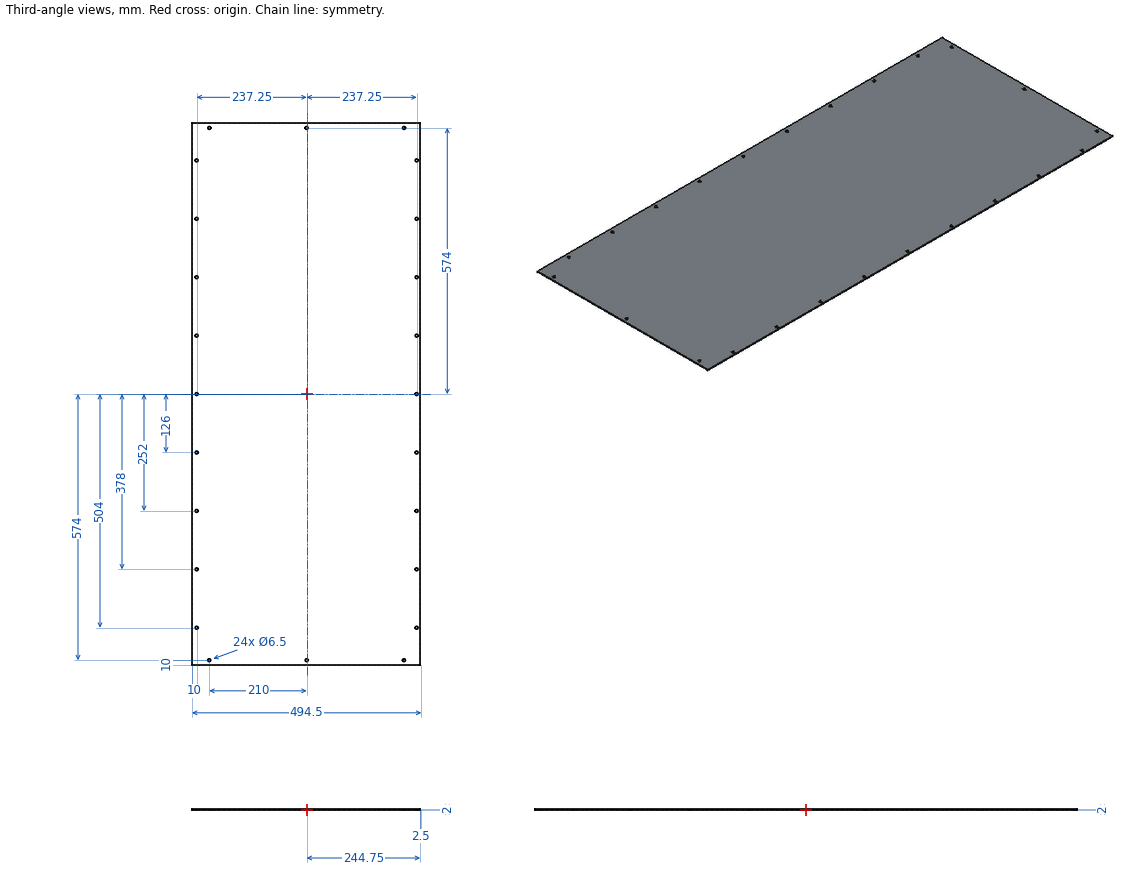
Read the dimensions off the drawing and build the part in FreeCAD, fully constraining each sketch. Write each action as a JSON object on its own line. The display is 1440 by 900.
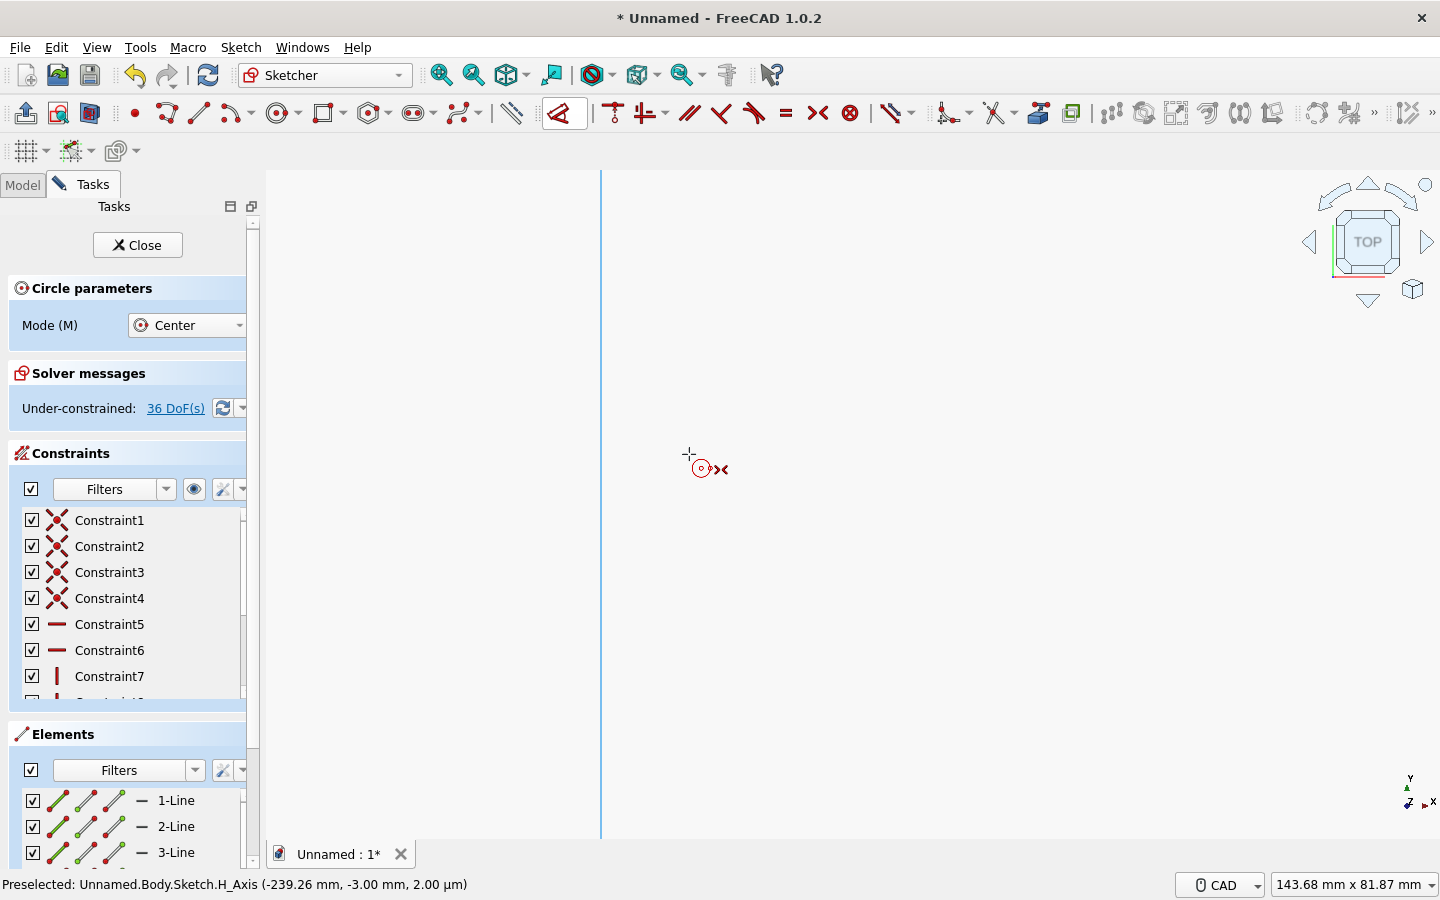
{"action": "scroll", "coordinate": [689, 454], "scroll_direction": "down", "scroll_amount": 15}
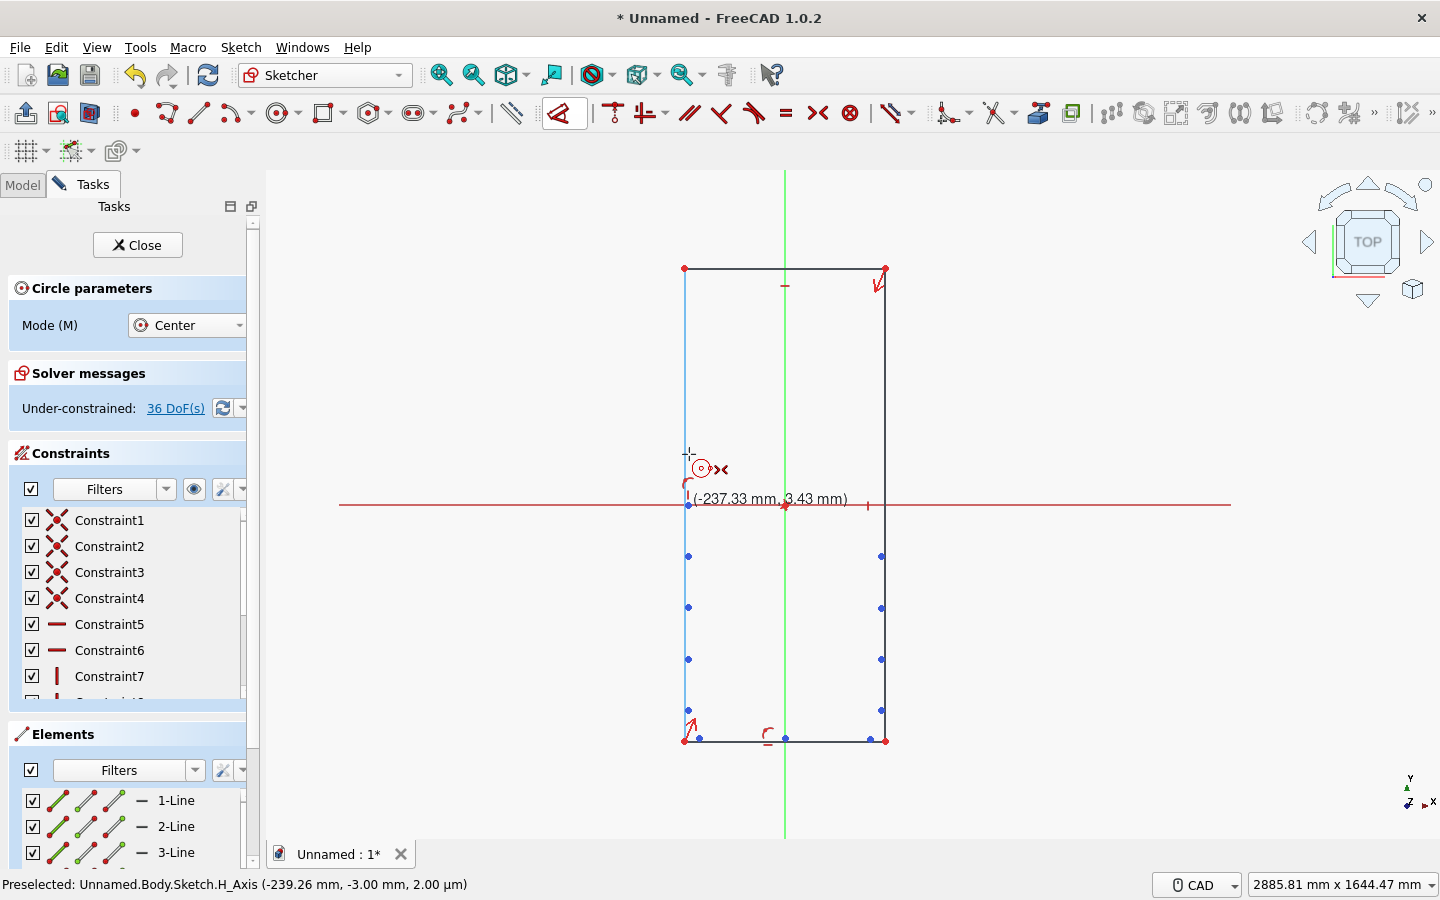
{"action": "scroll", "coordinate": [689, 454], "scroll_direction": "up", "scroll_amount": 7}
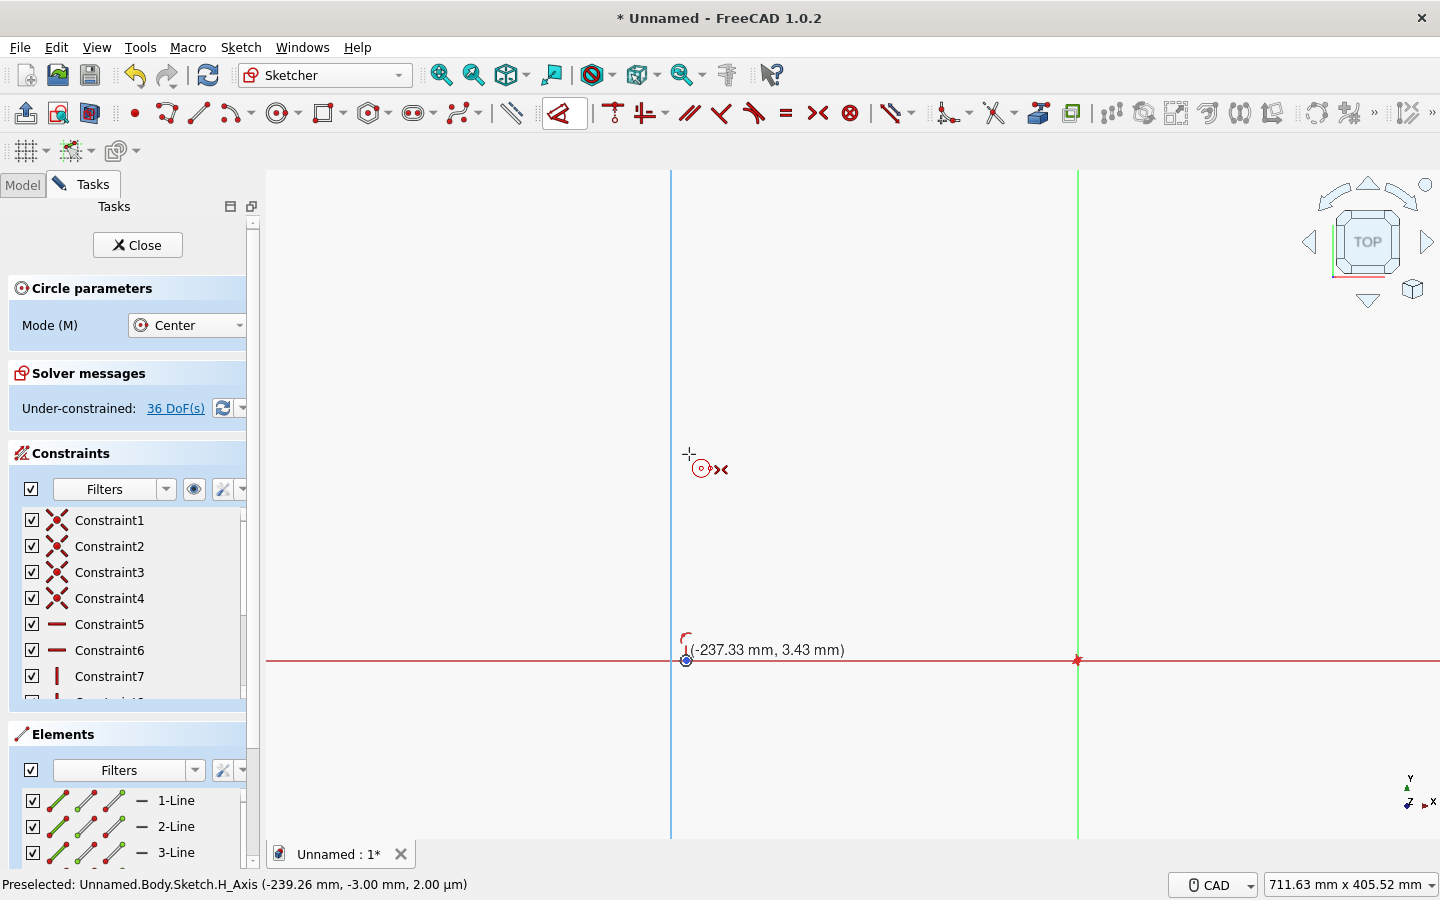
{"action": "left_click", "coordinate": [686, 453]}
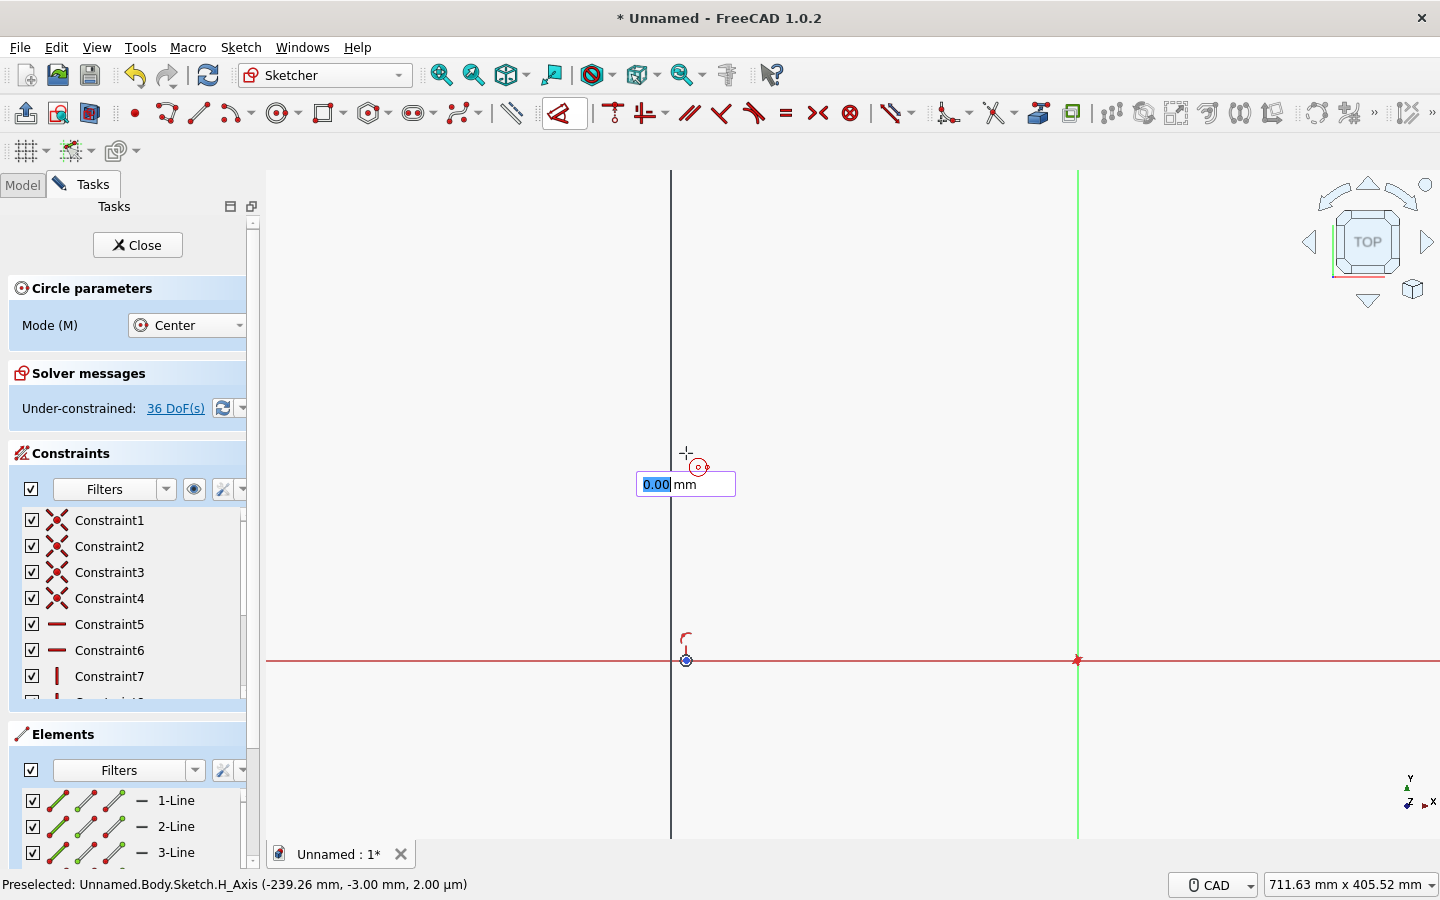
{"action": "scroll", "coordinate": [690, 449], "scroll_direction": "up", "scroll_amount": 6}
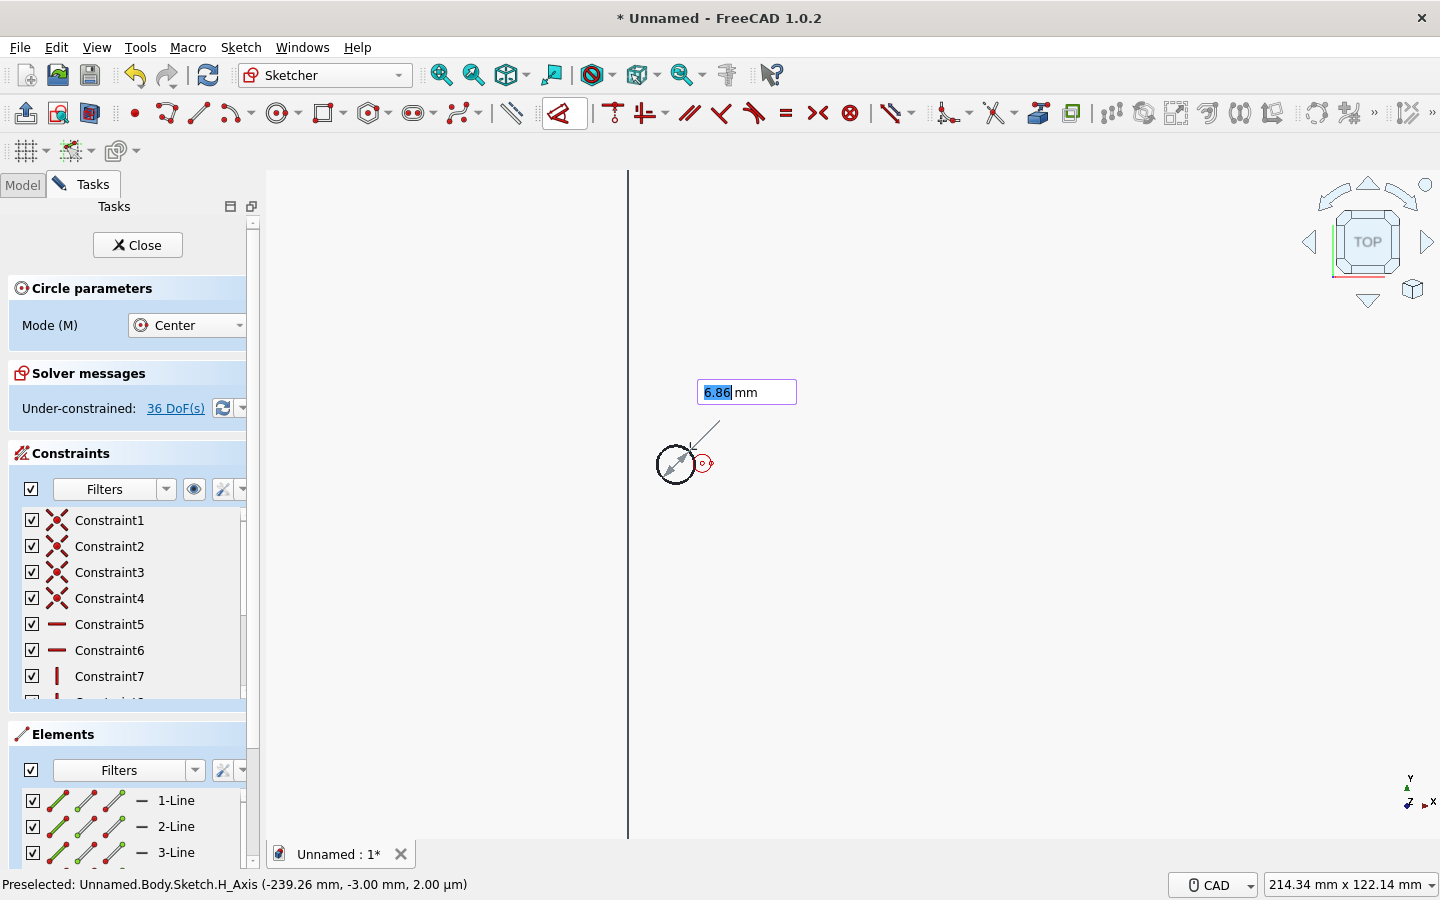
{"action": "left_click", "coordinate": [689, 448]}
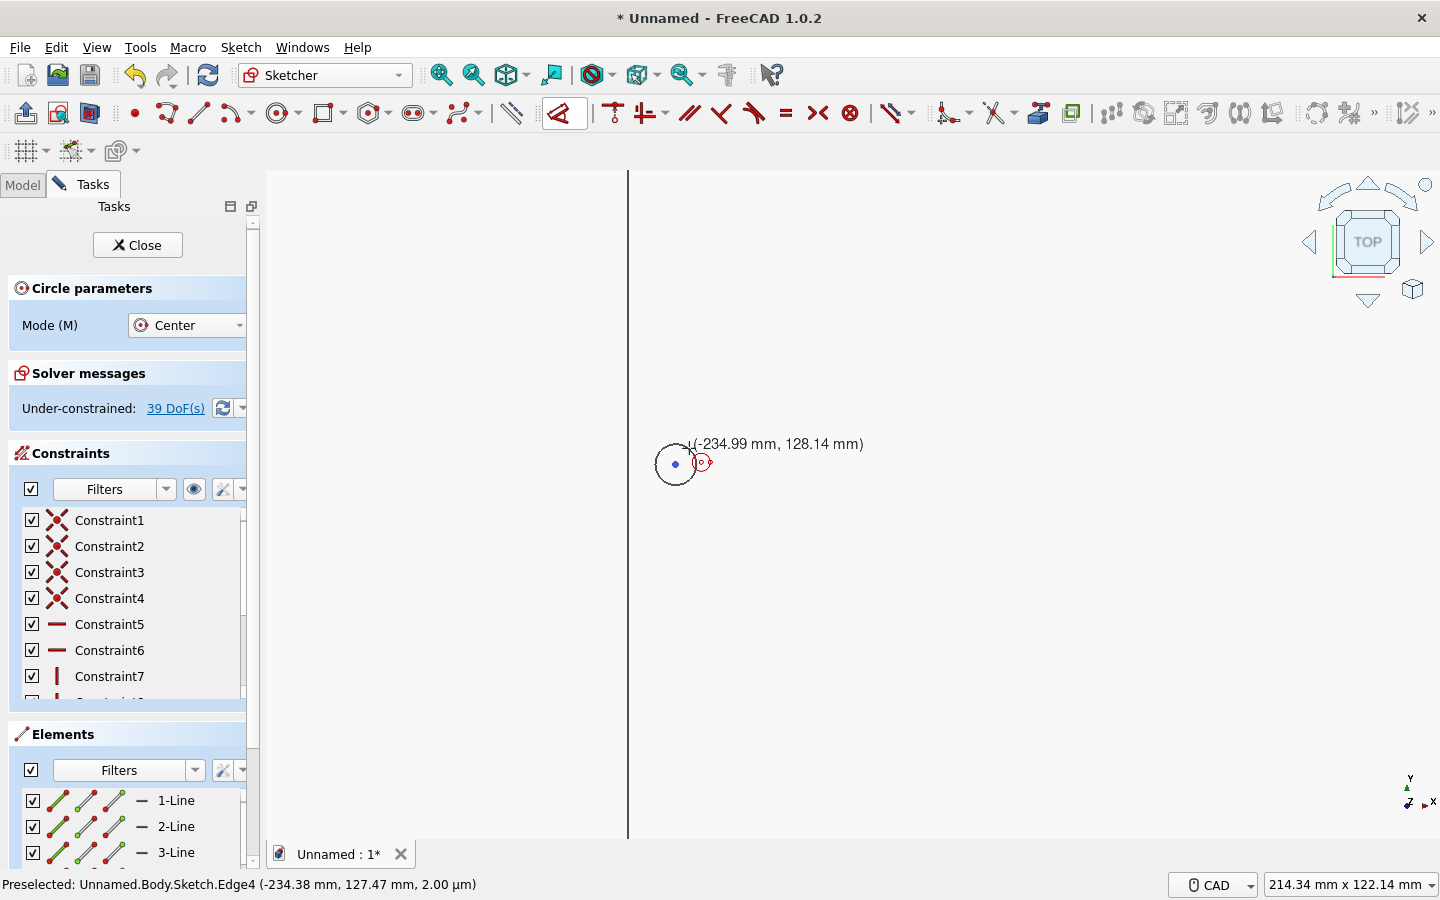
{"action": "scroll", "coordinate": [689, 453], "scroll_direction": "down", "scroll_amount": 13}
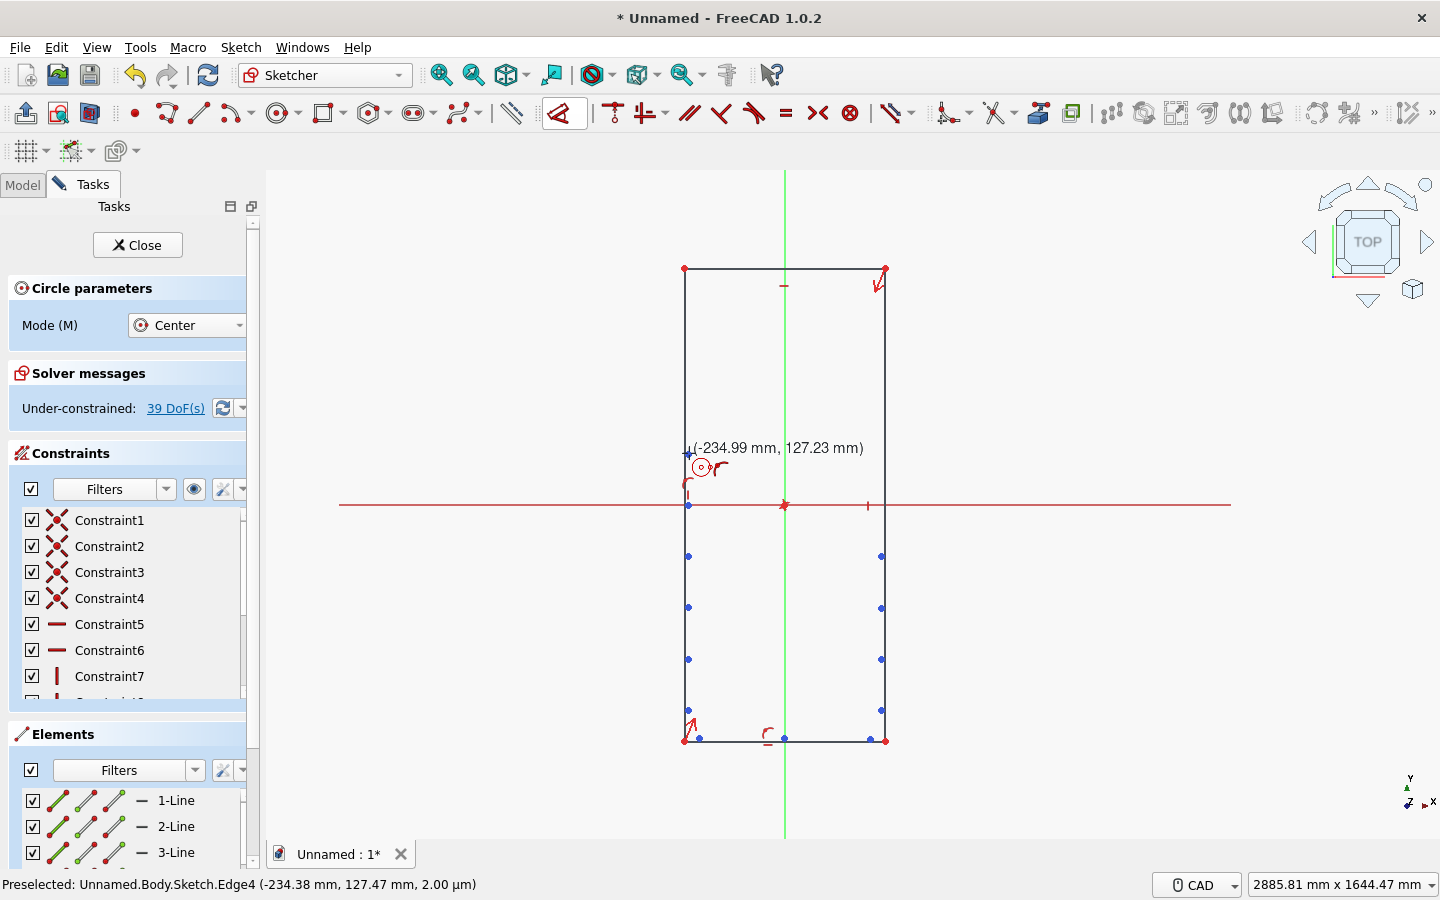
{"action": "scroll", "coordinate": [688, 403], "scroll_direction": "up", "scroll_amount": 15}